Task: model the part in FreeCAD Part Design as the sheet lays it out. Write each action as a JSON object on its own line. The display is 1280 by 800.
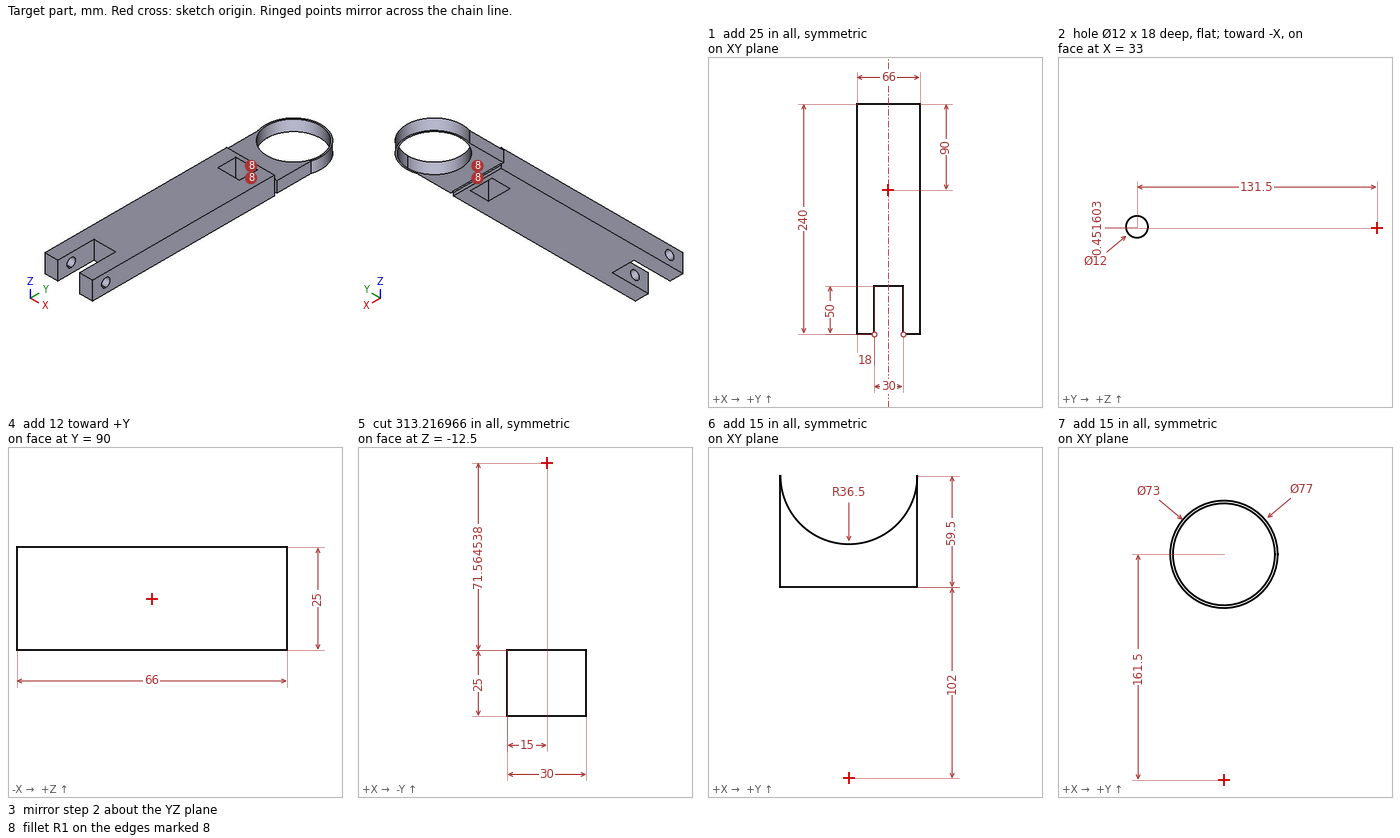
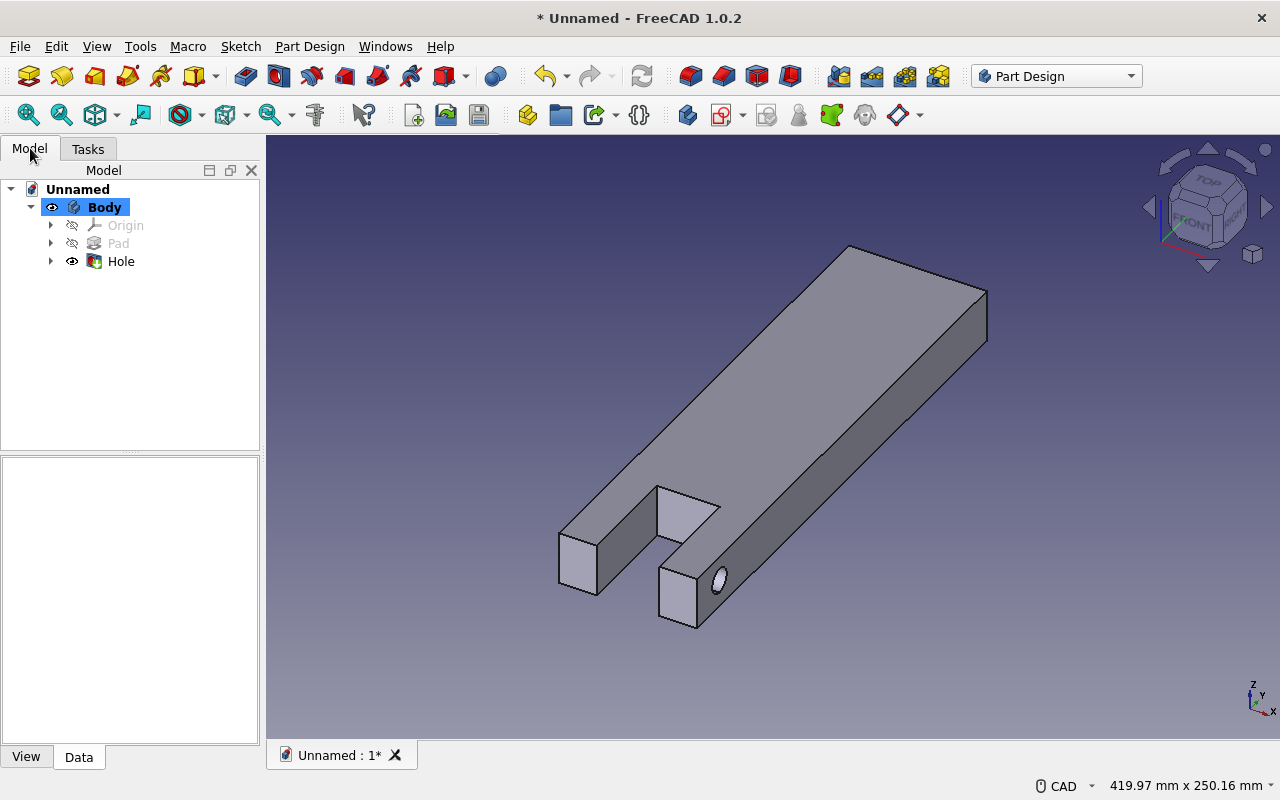
{"action": "left_click", "coordinate": [117, 261]}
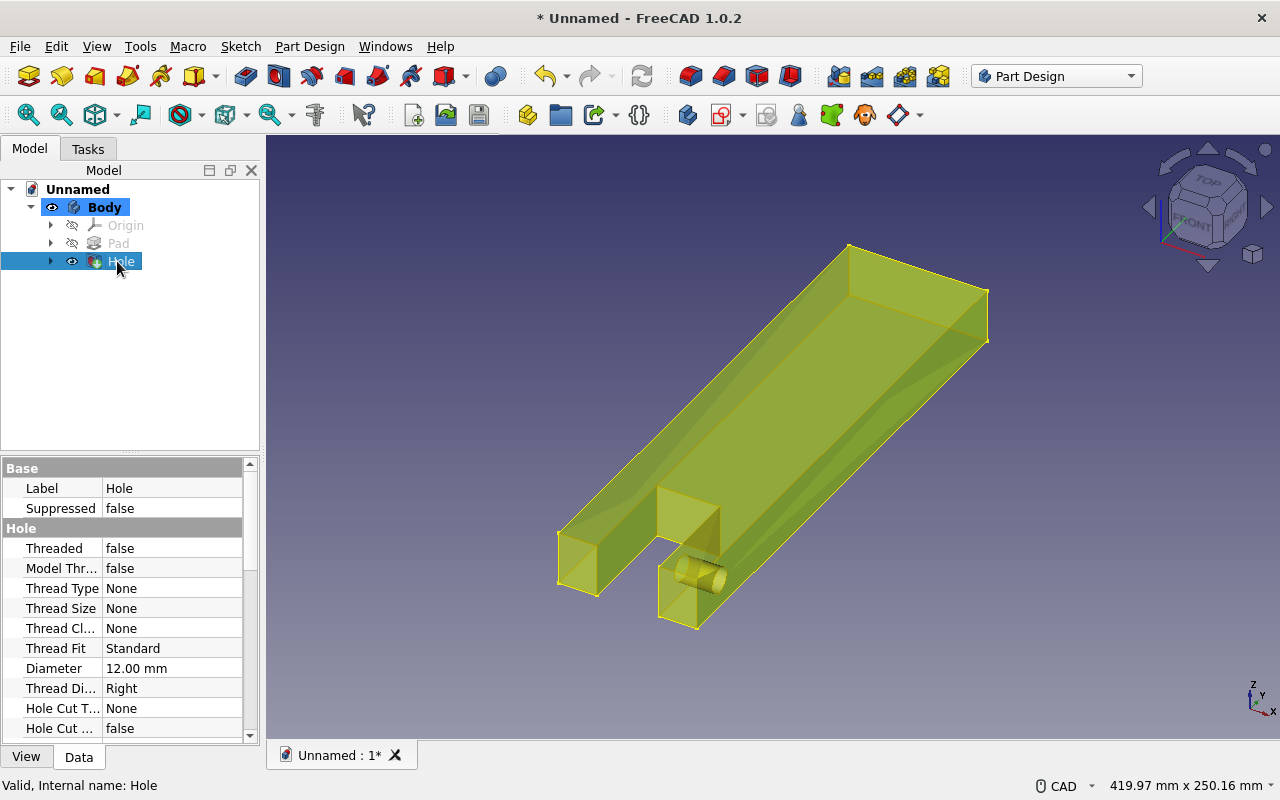
{"action": "left_click", "coordinate": [839, 76]}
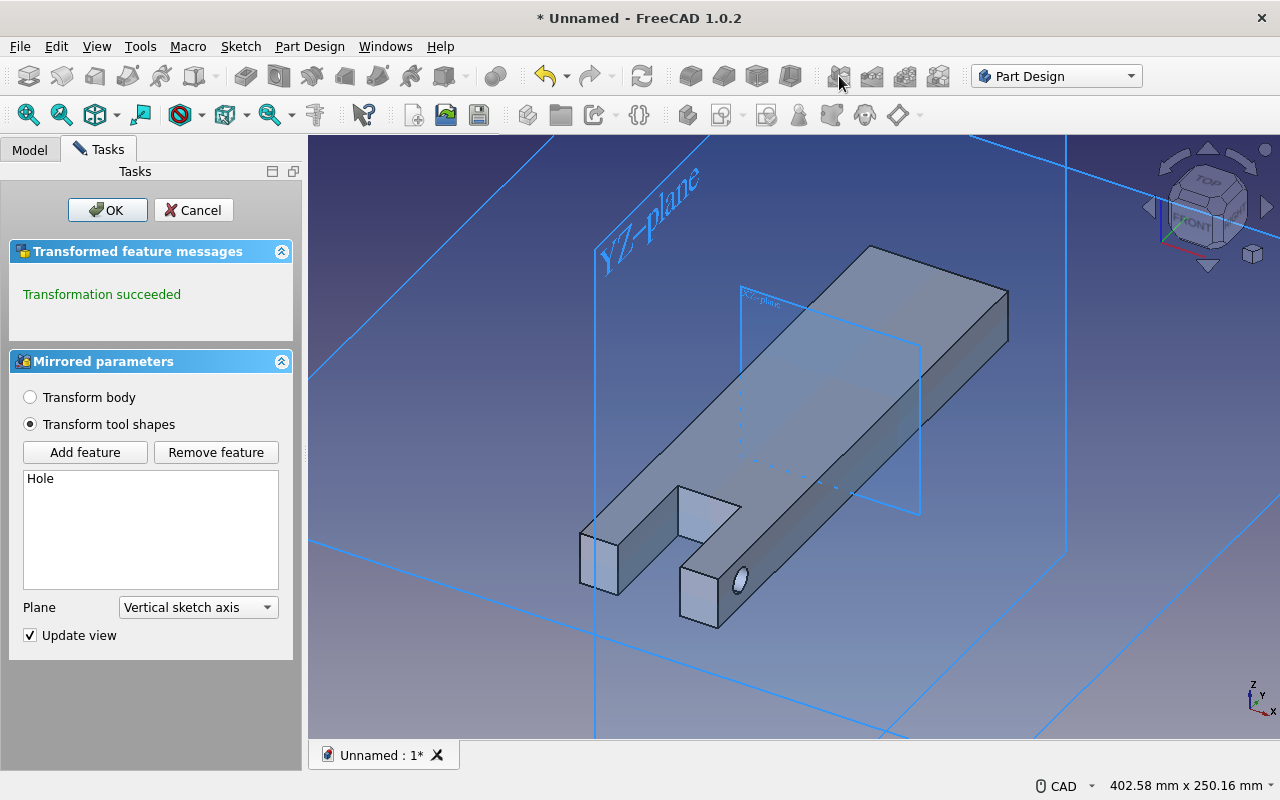
{"action": "left_click", "coordinate": [199, 608]}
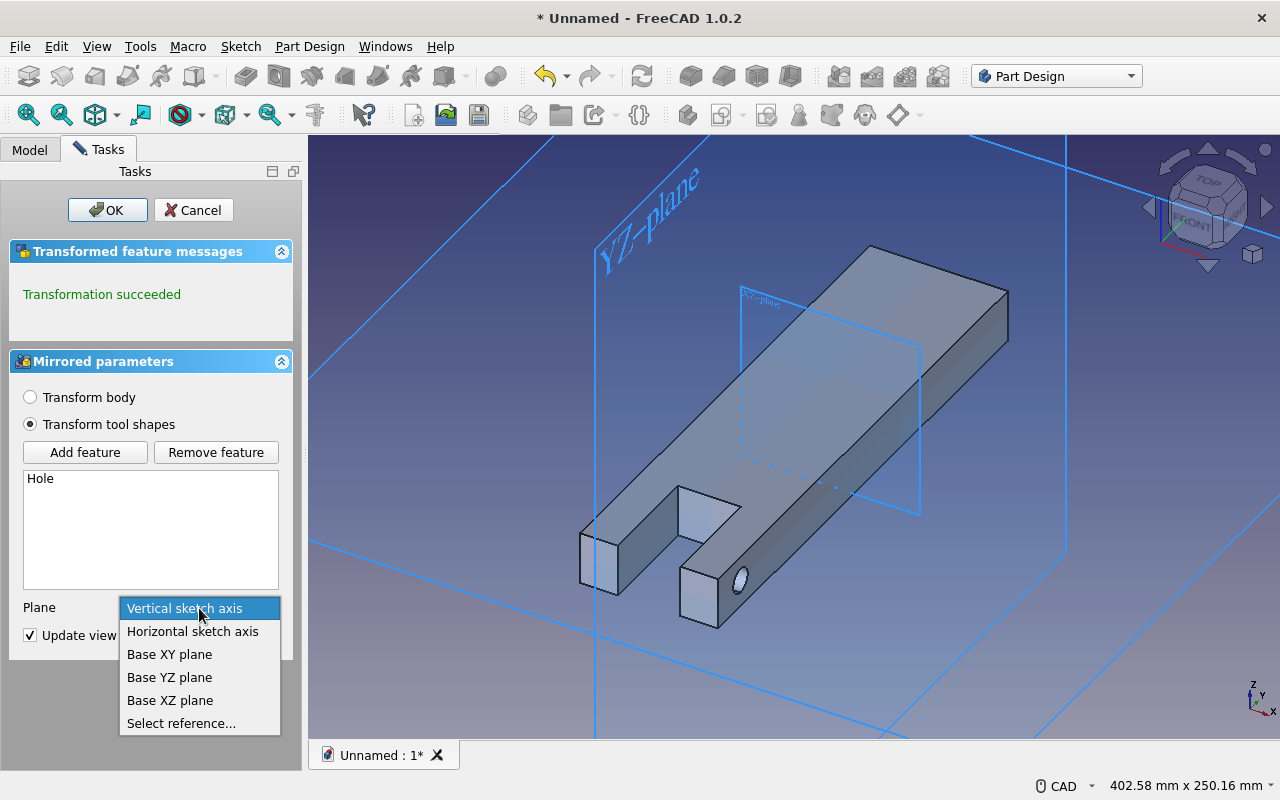
{"action": "left_click", "coordinate": [198, 678]}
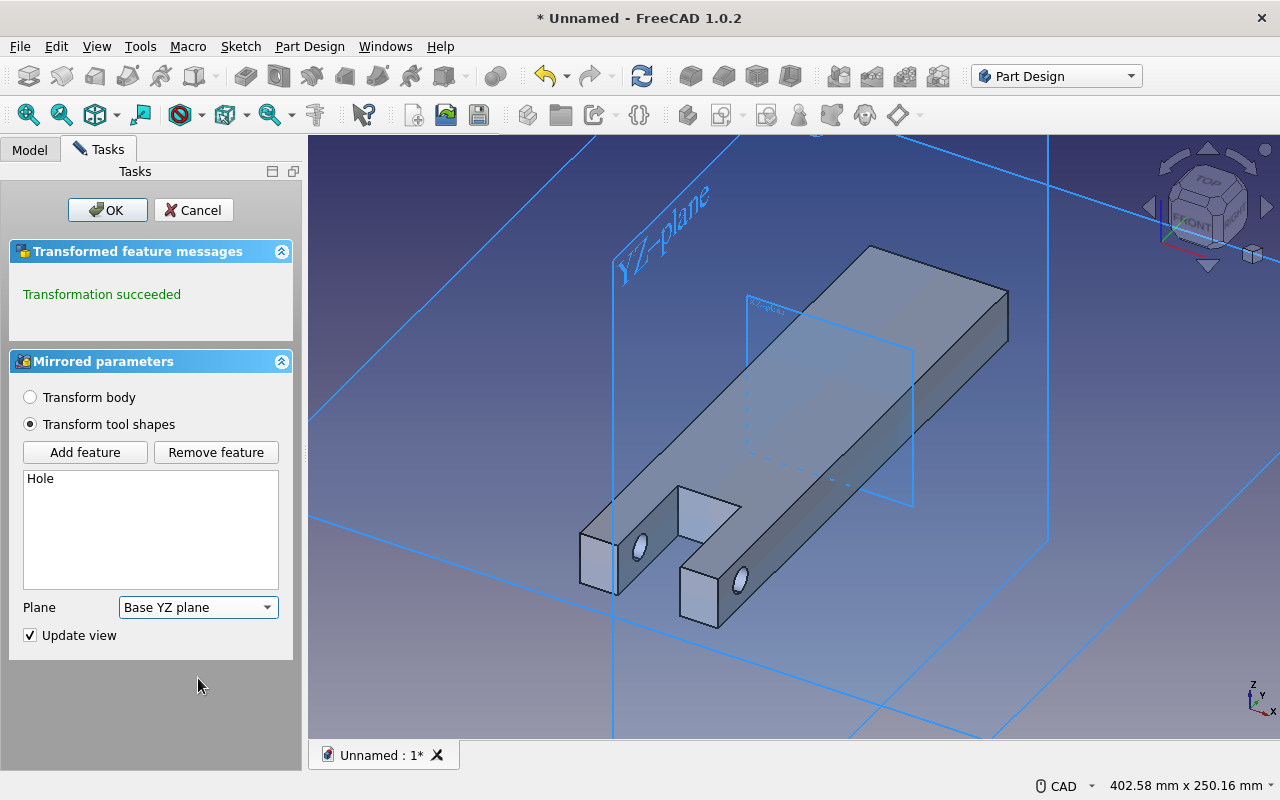
{"action": "left_click", "coordinate": [108, 210]}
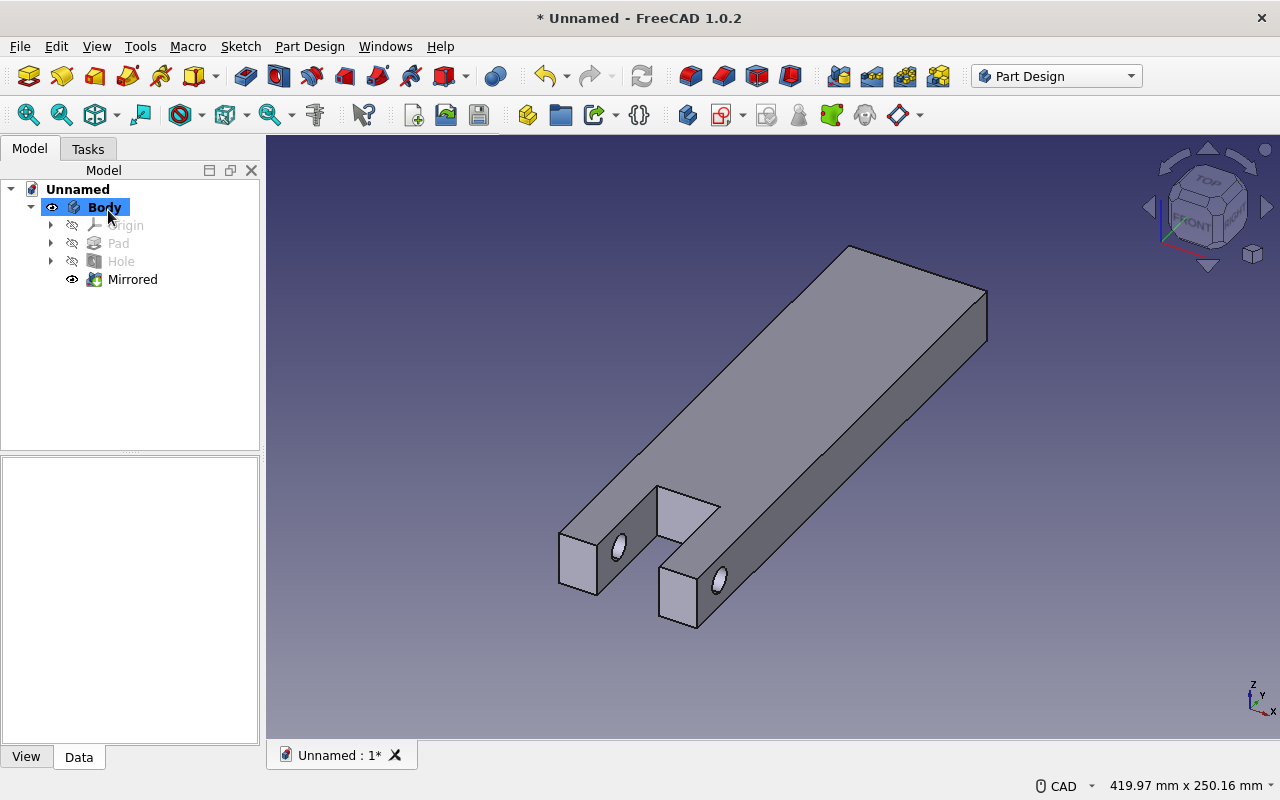
{"action": "key", "text": "4"}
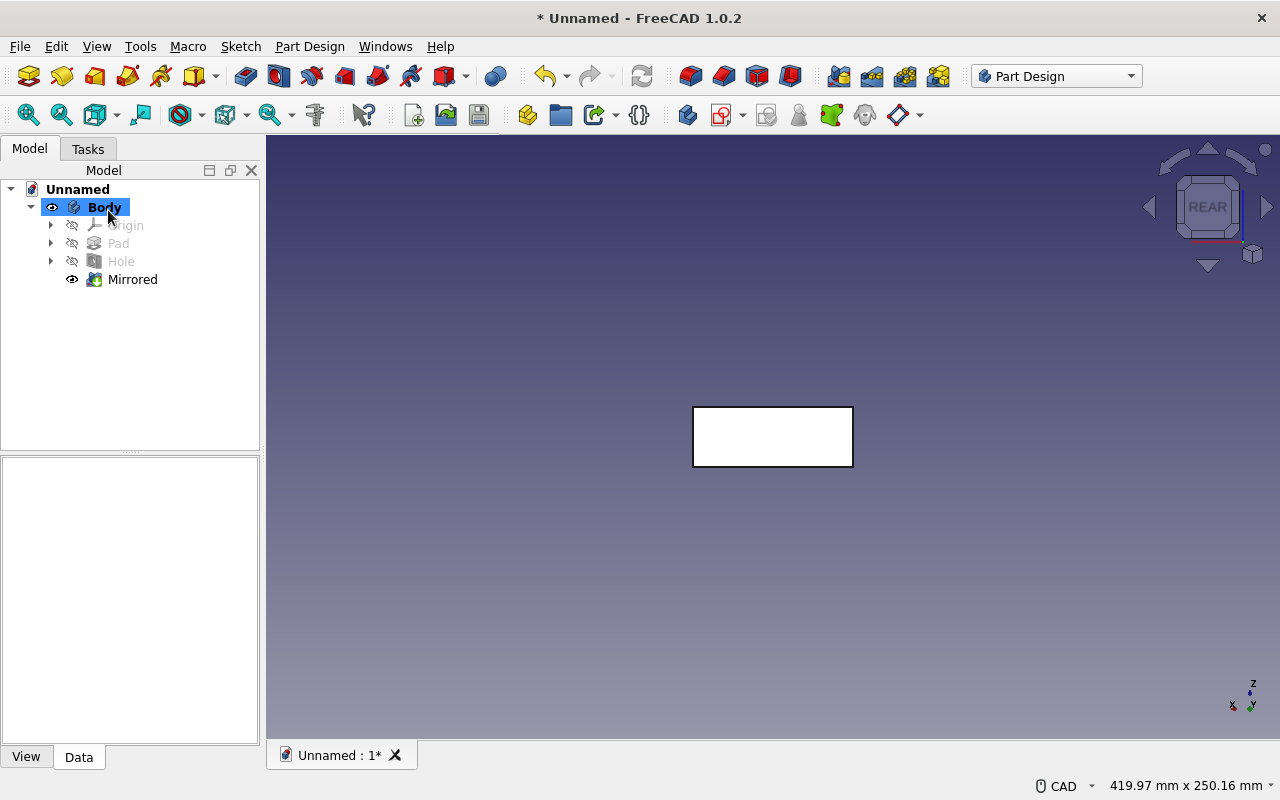
{"action": "key", "text": "v f"}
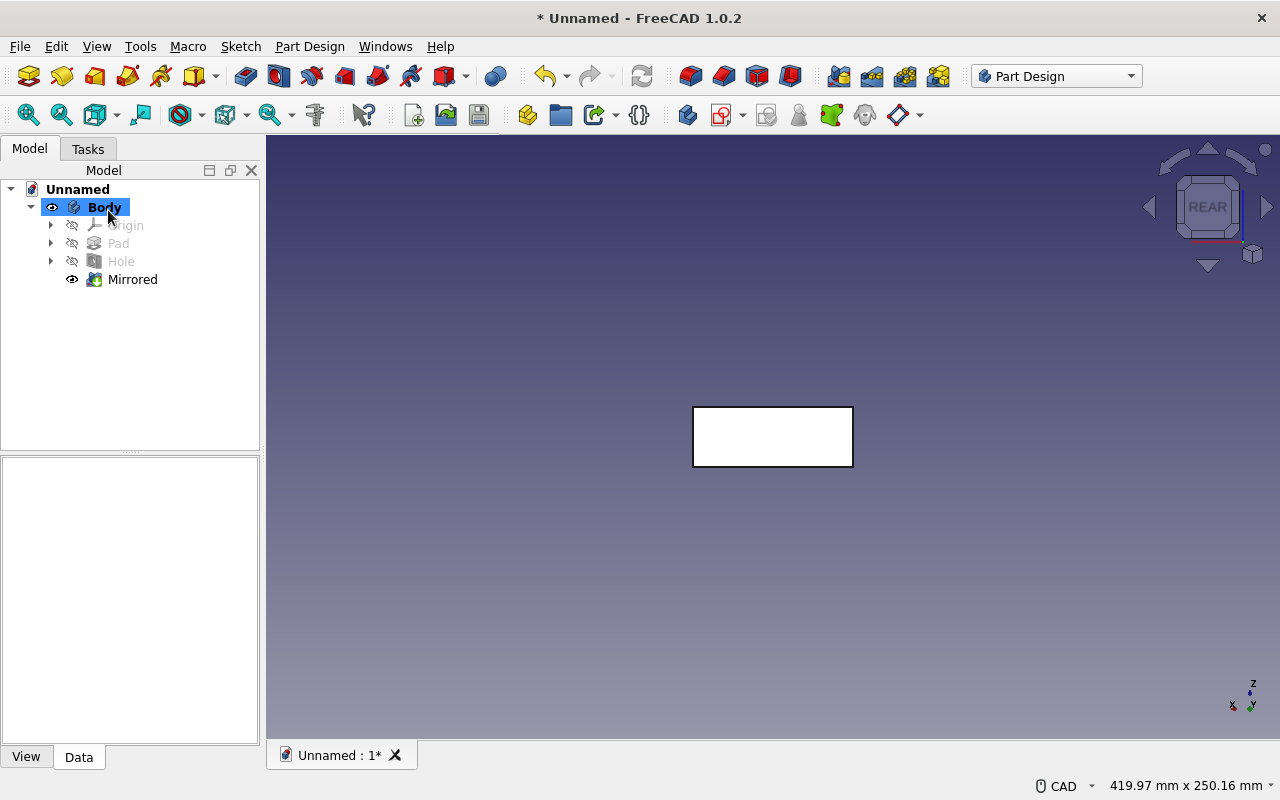
{"action": "left_click", "coordinate": [727, 436]}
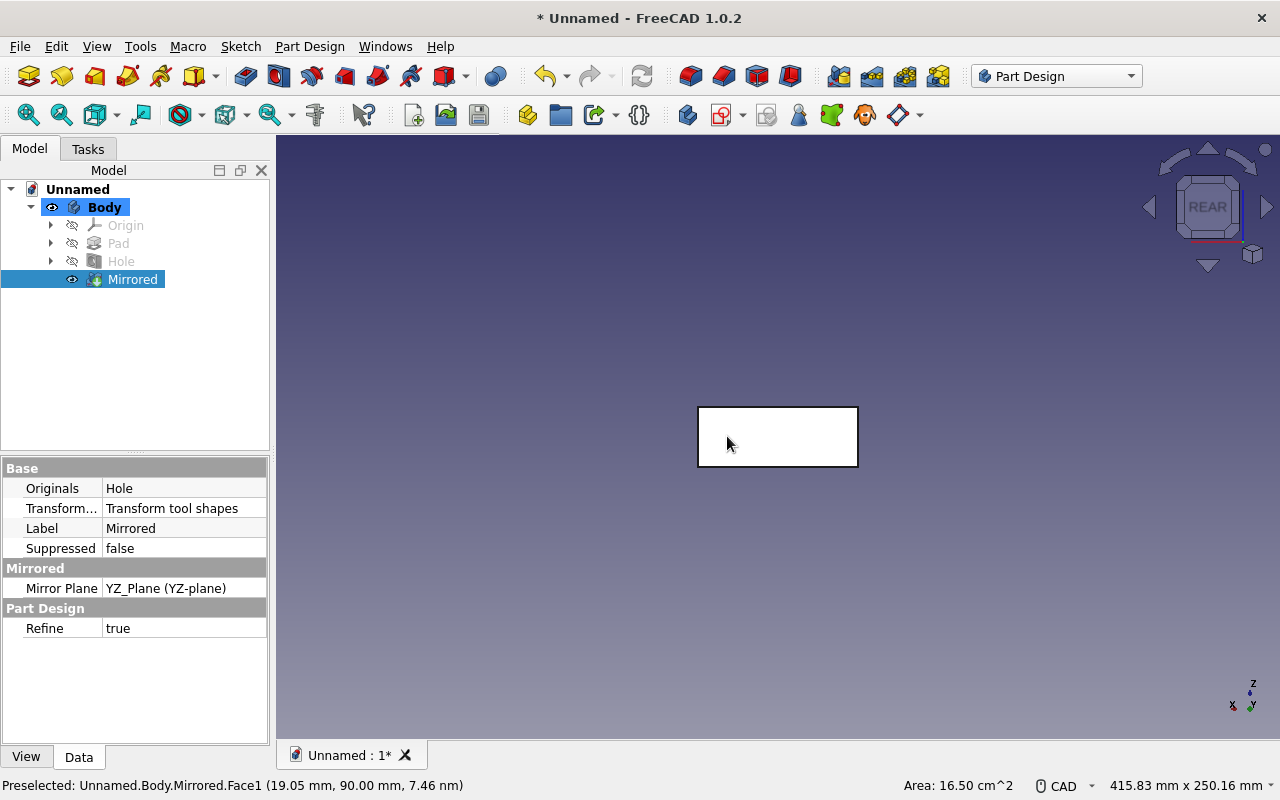
{"action": "left_click", "coordinate": [720, 116]}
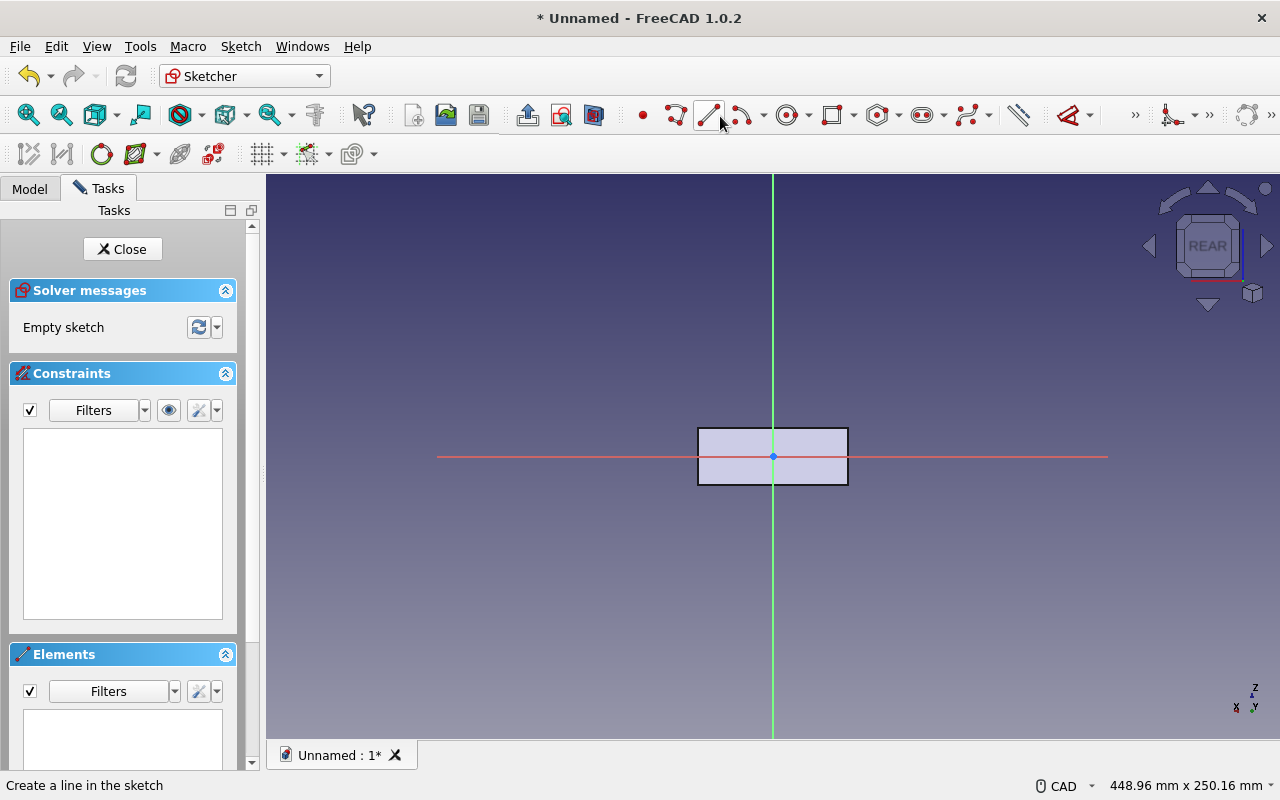
{"action": "scroll", "coordinate": [795, 456], "scroll_direction": "up", "scroll_amount": 7}